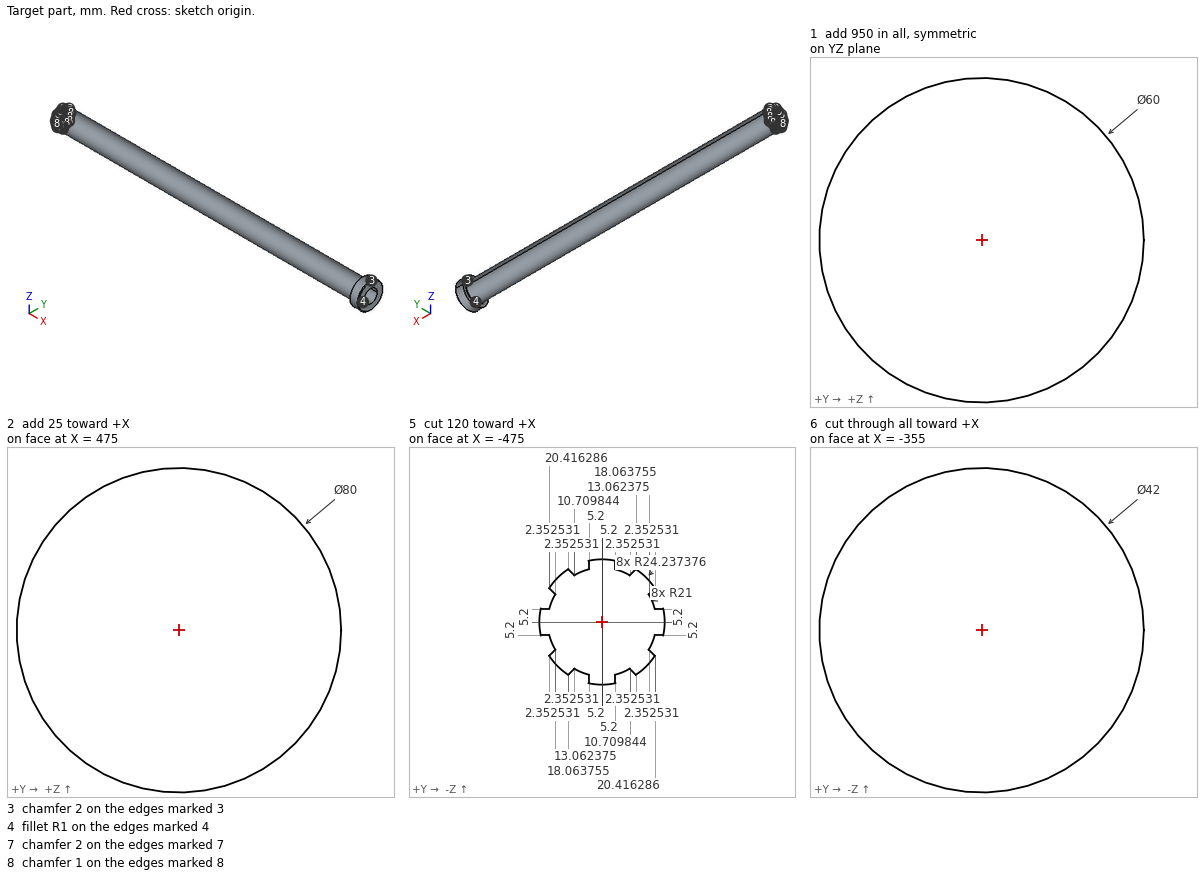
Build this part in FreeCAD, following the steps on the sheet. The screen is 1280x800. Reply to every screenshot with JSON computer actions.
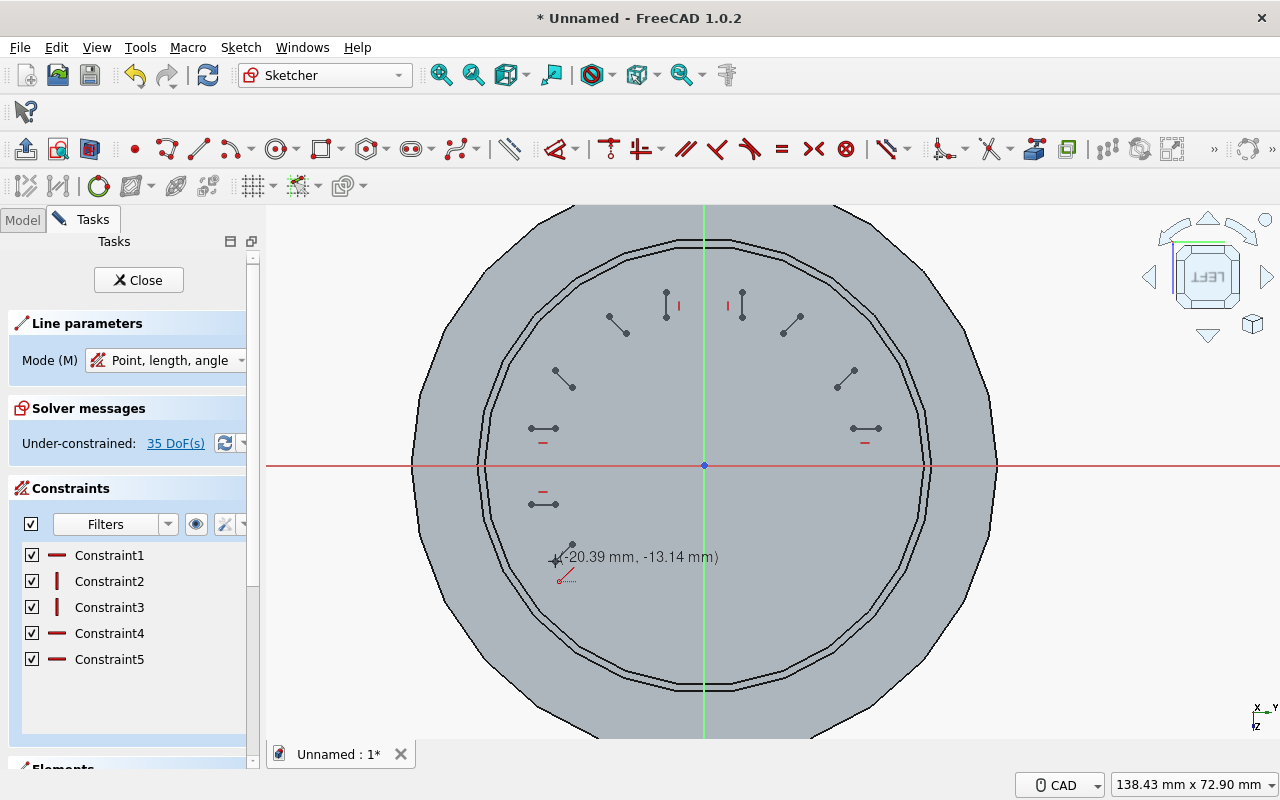
{"action": "left_click", "coordinate": [609, 615]}
{"action": "left_click", "coordinate": [626, 598]}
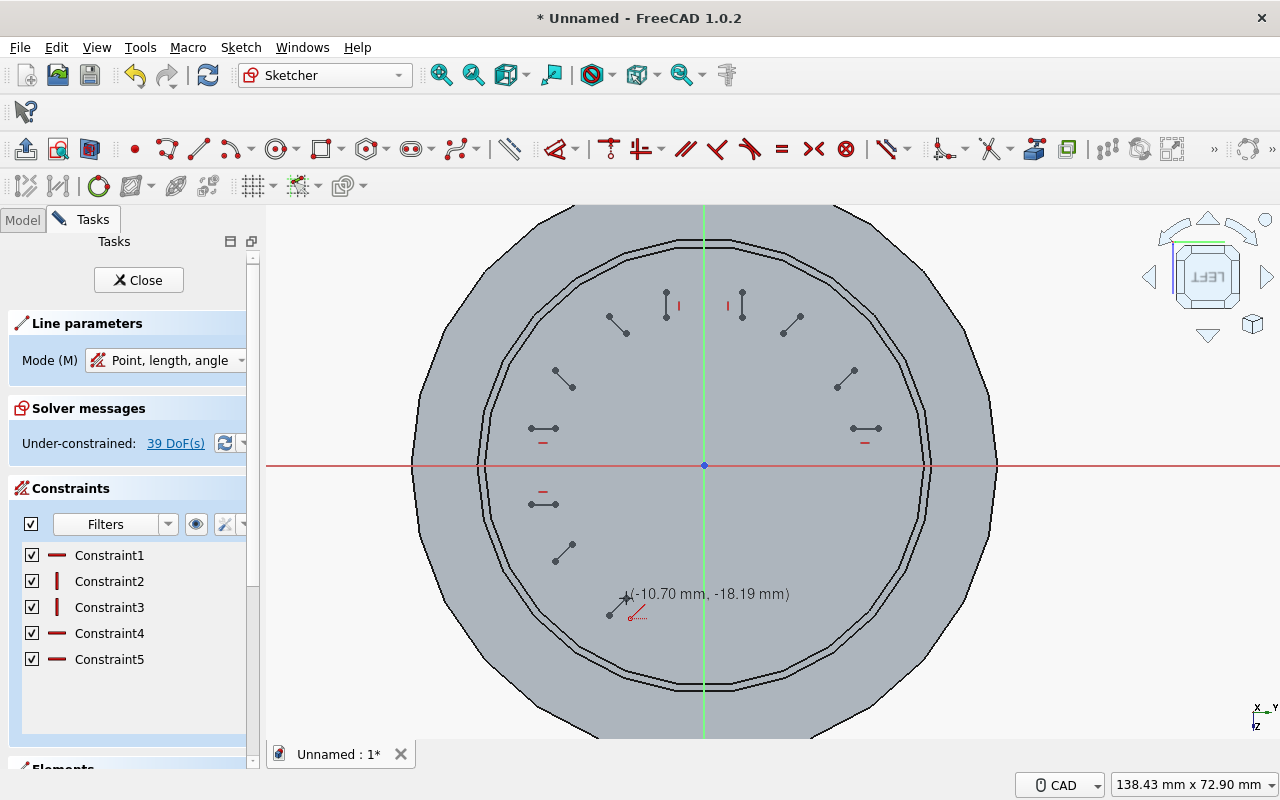
{"action": "left_click", "coordinate": [666, 615]}
{"action": "left_click", "coordinate": [666, 639]}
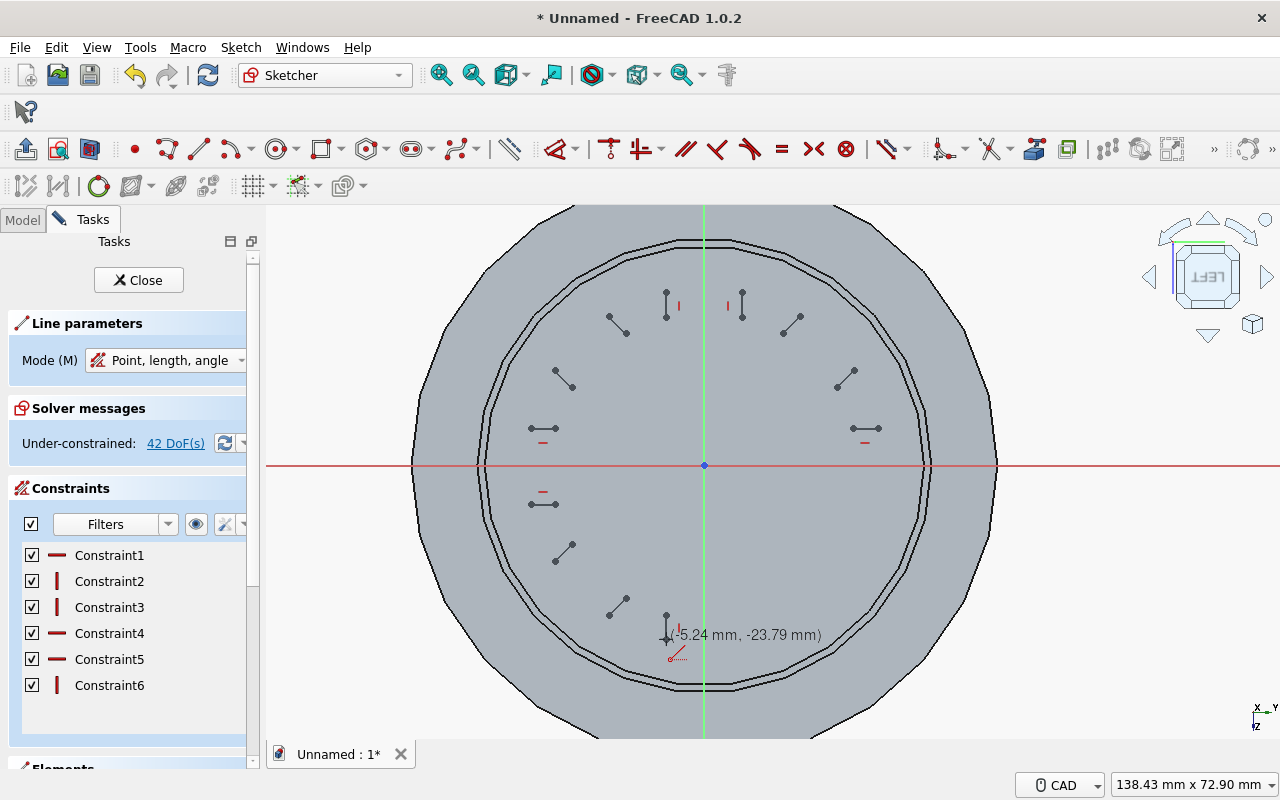
{"action": "left_click", "coordinate": [742, 639]}
{"action": "left_click", "coordinate": [742, 615]}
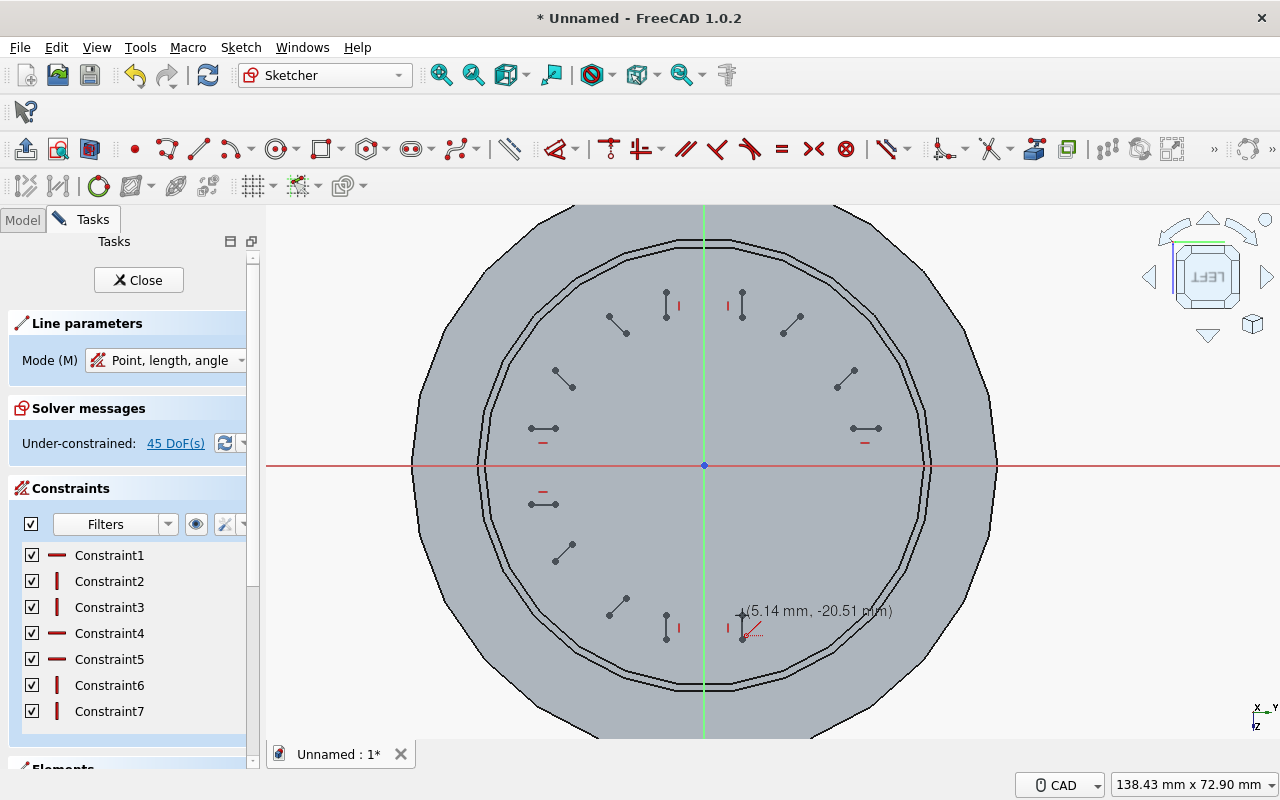
{"action": "left_click", "coordinate": [783, 598]}
{"action": "left_click", "coordinate": [800, 615]}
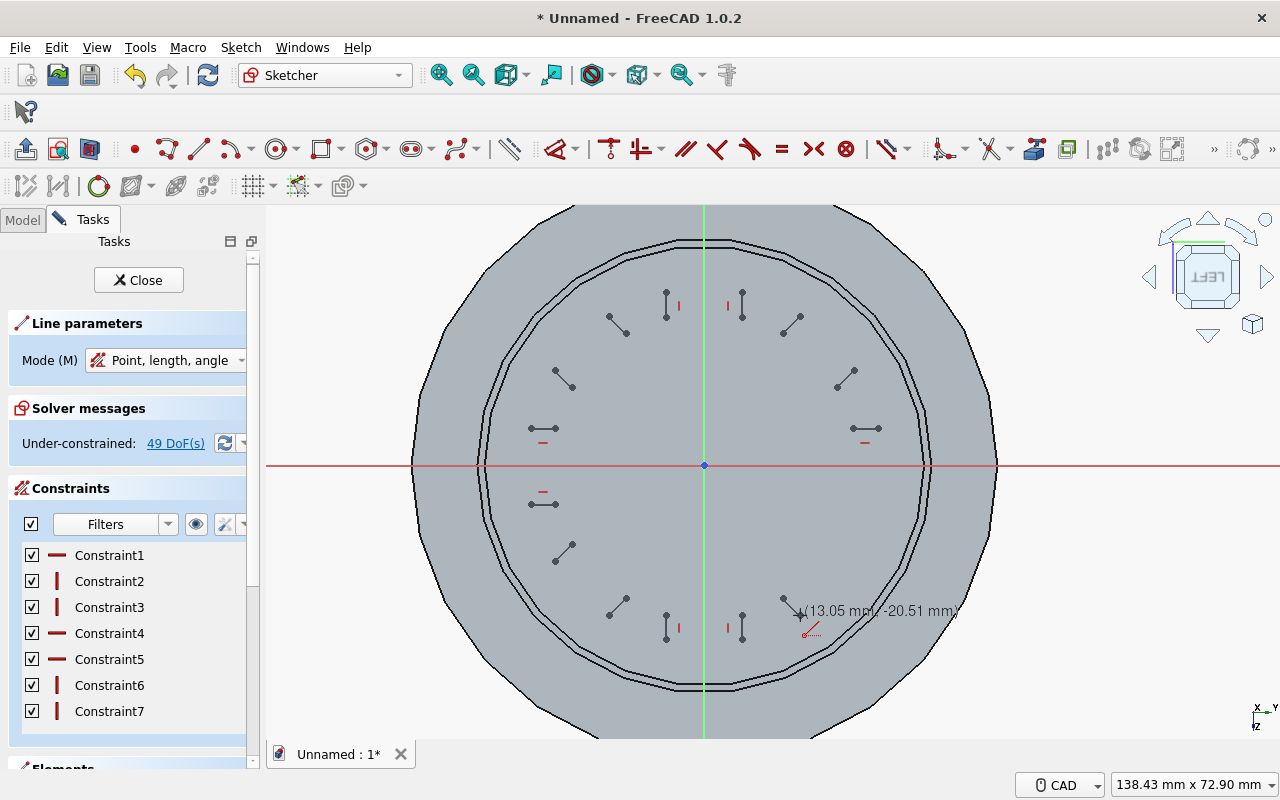
{"action": "left_click", "coordinate": [854, 561]}
{"action": "left_click", "coordinate": [837, 544]}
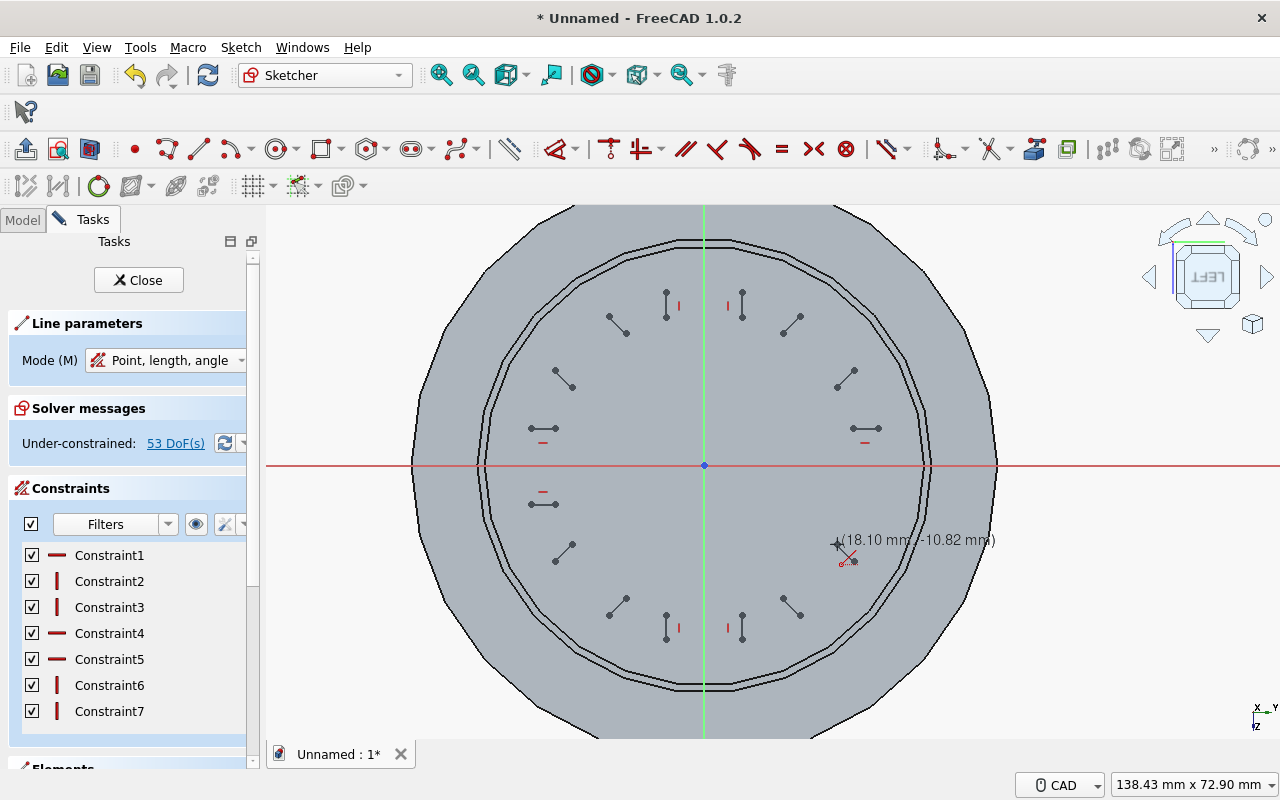
{"action": "left_click", "coordinate": [853, 504]}
{"action": "left_click", "coordinate": [878, 504]}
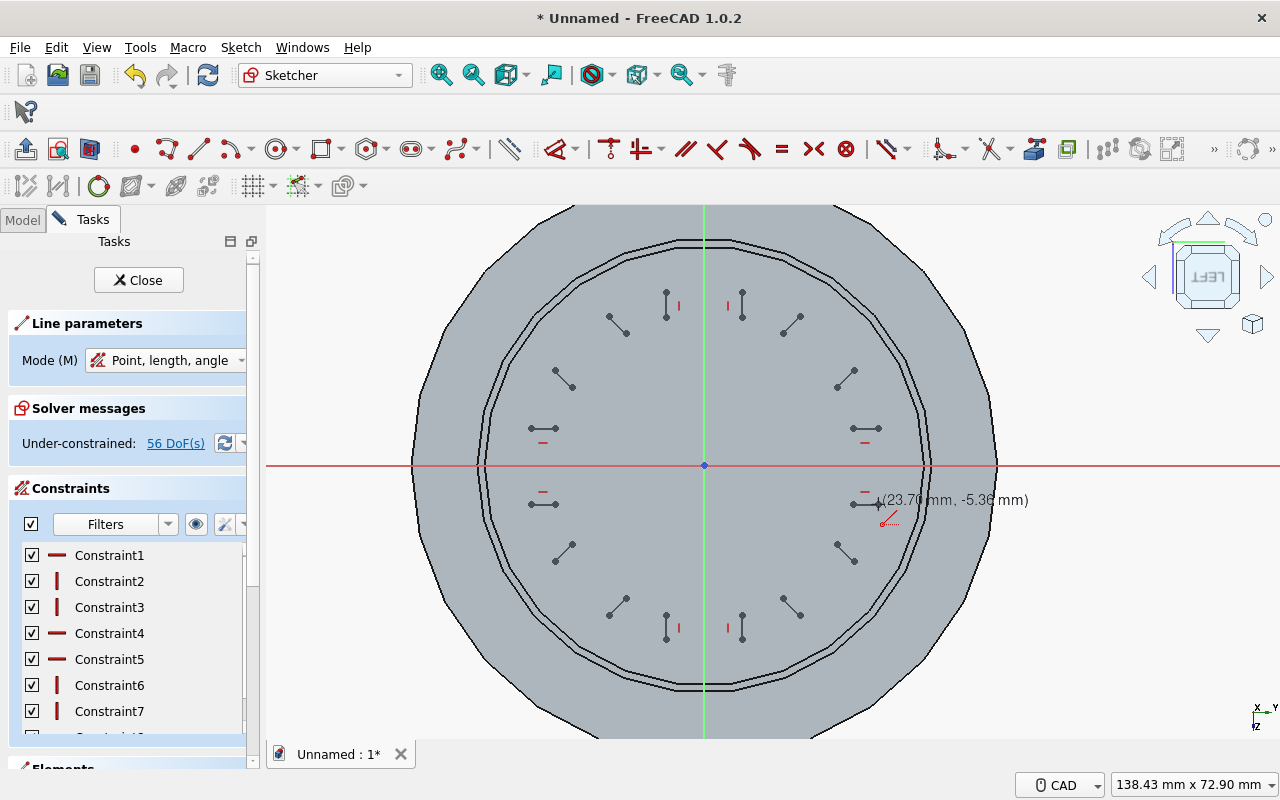
{"action": "key", "text": "g 3 a"}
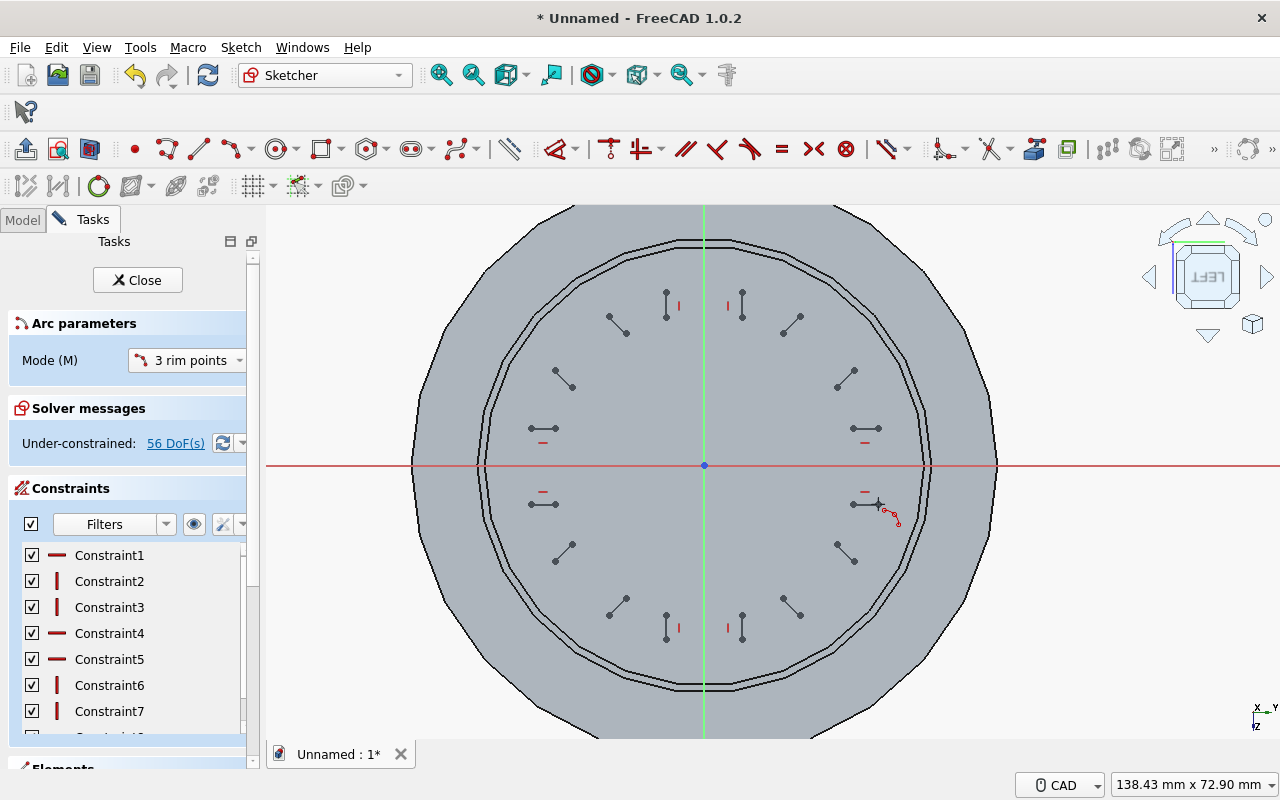
{"action": "scroll", "coordinate": [853, 428], "scroll_direction": "up", "scroll_amount": 2}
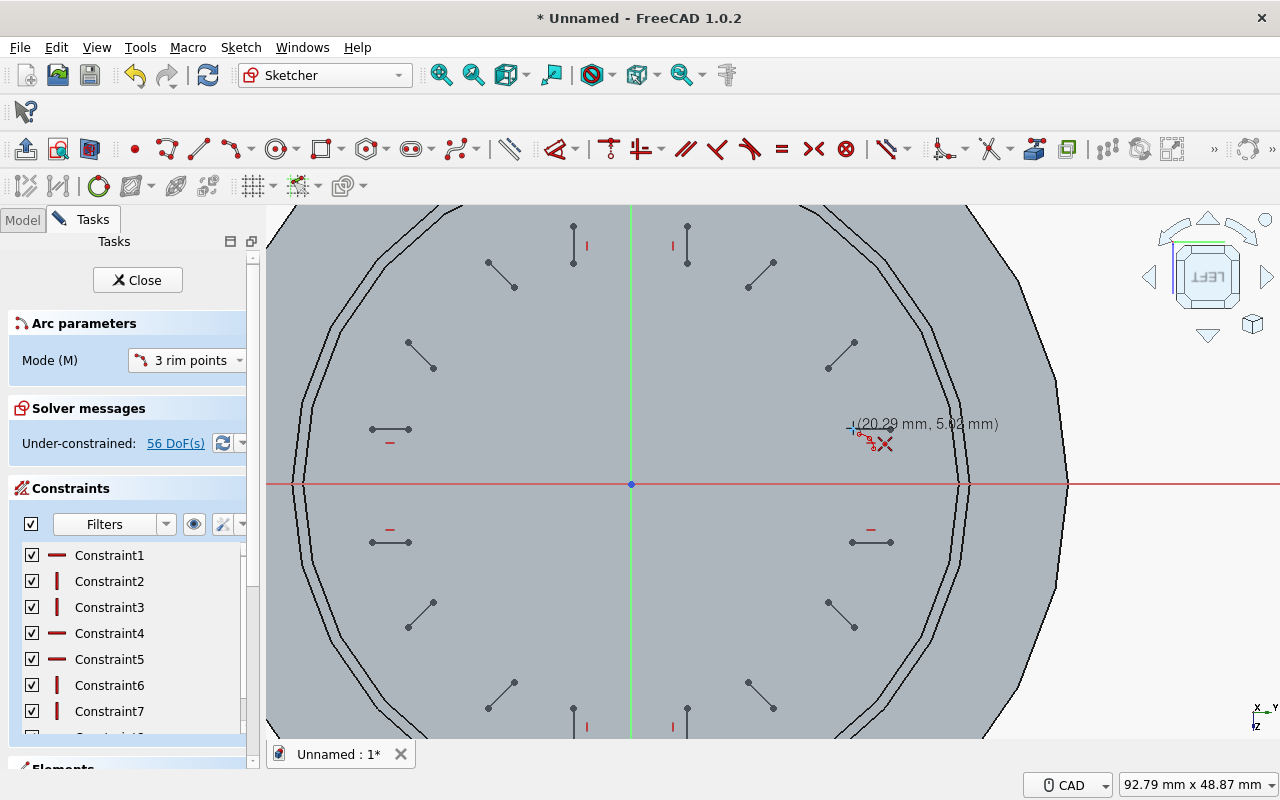
{"action": "left_click", "coordinate": [853, 429]}
{"action": "left_click", "coordinate": [829, 368]}